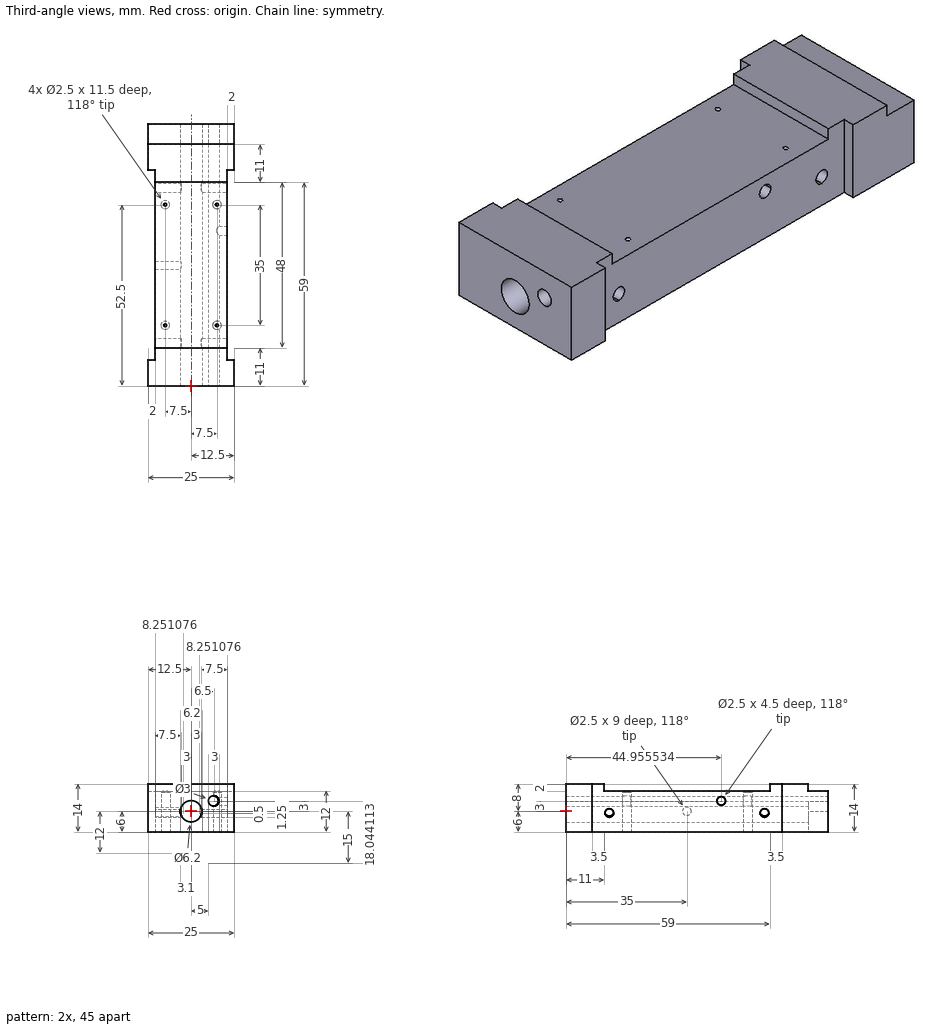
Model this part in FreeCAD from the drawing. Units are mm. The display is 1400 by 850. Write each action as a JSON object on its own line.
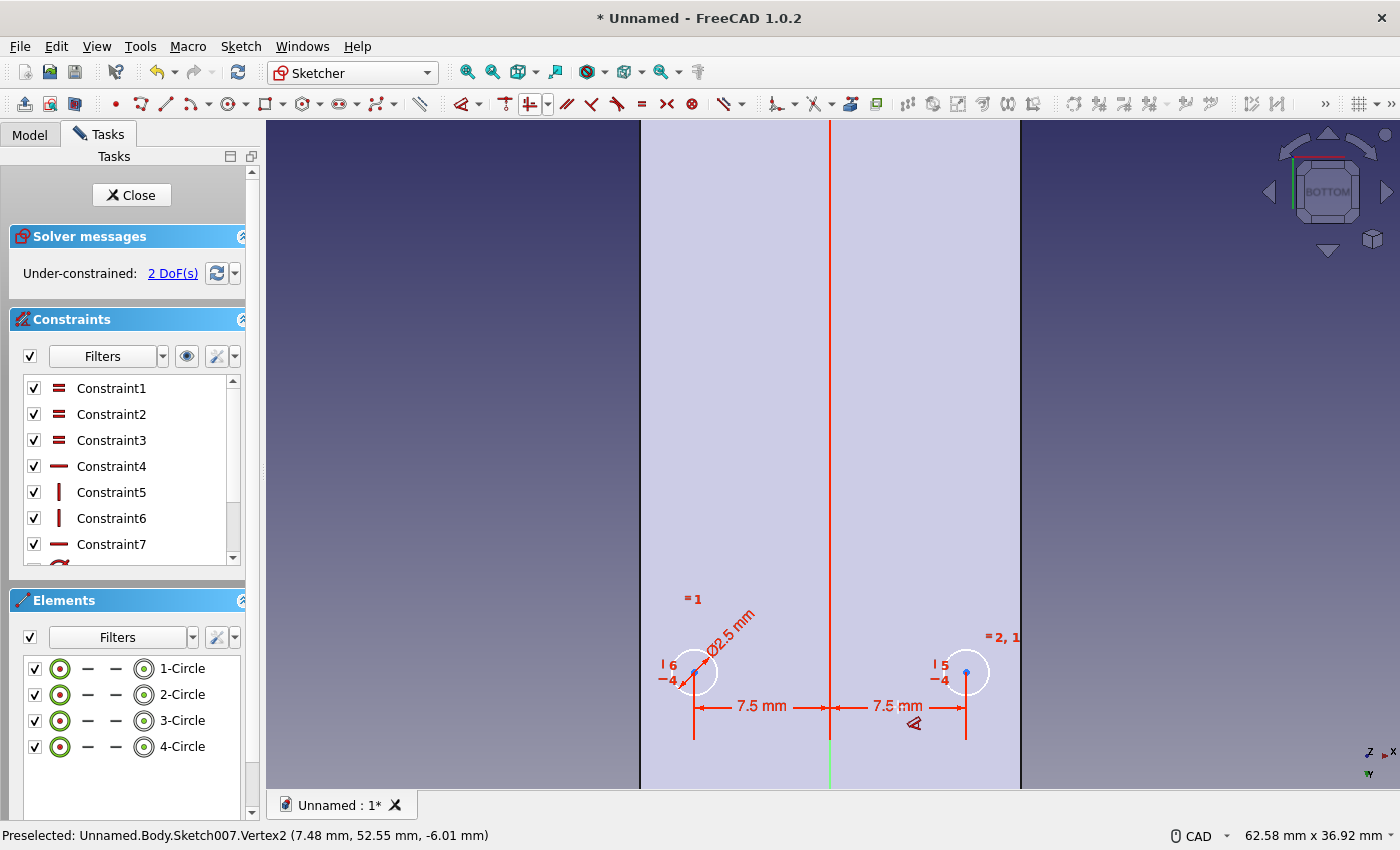
{"action": "left_click", "coordinate": [966, 673]}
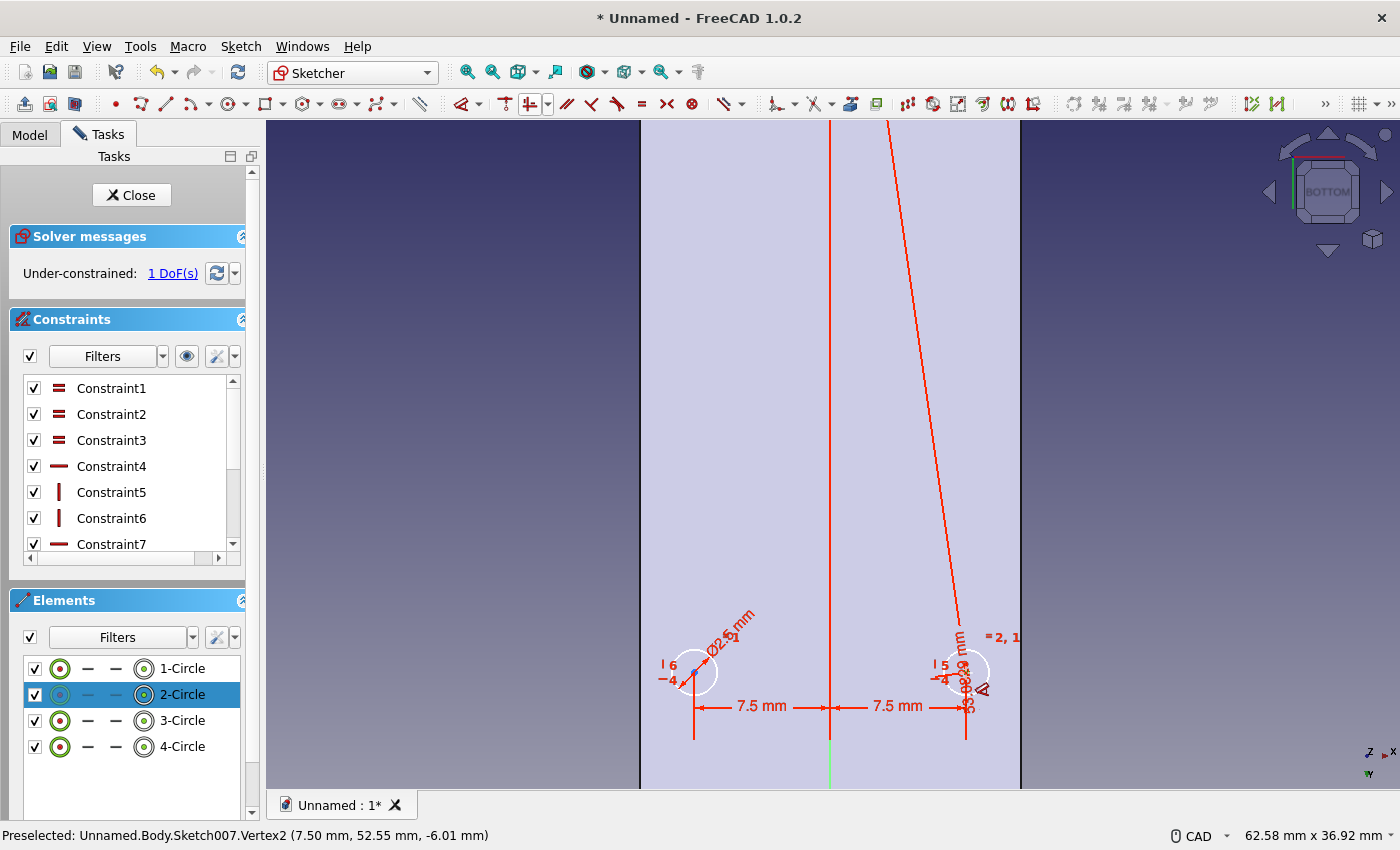
{"action": "scroll", "coordinate": [711, 656], "scroll_direction": "down", "scroll_amount": 4}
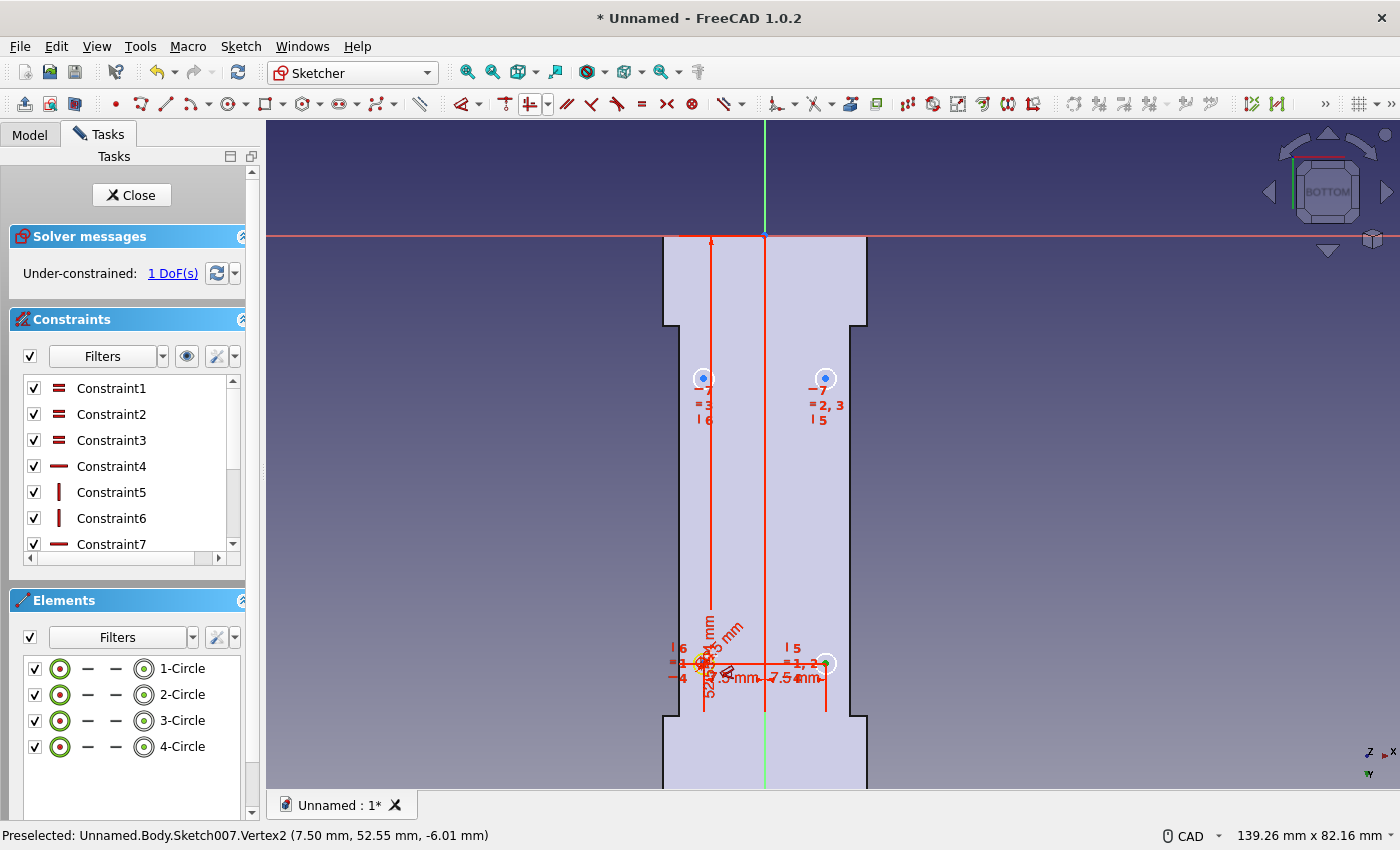
{"action": "left_click", "coordinate": [826, 379]}
{"action": "left_click", "coordinate": [860, 521]}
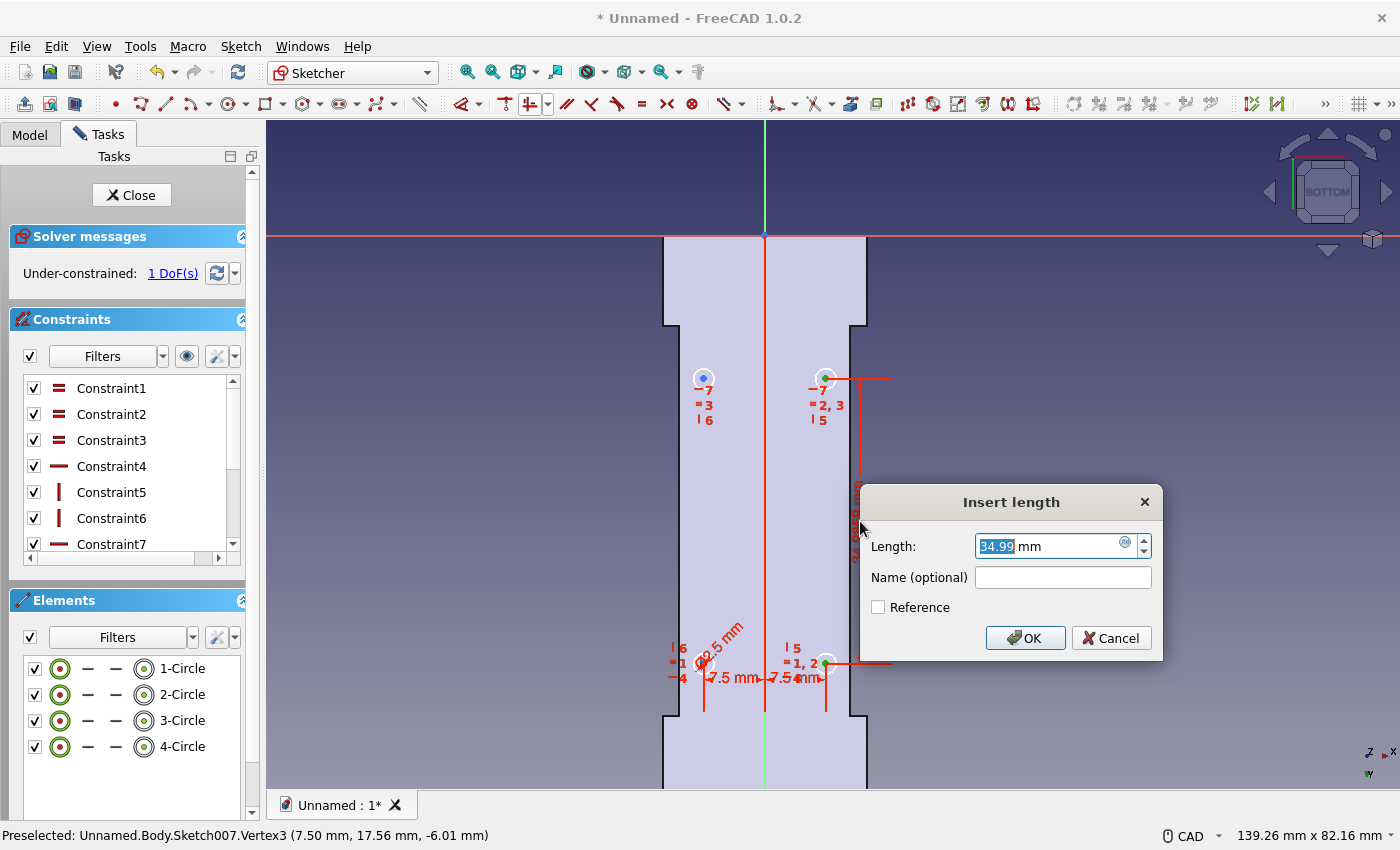
{"action": "type", "text": "35"}
{"action": "key", "text": "Return"}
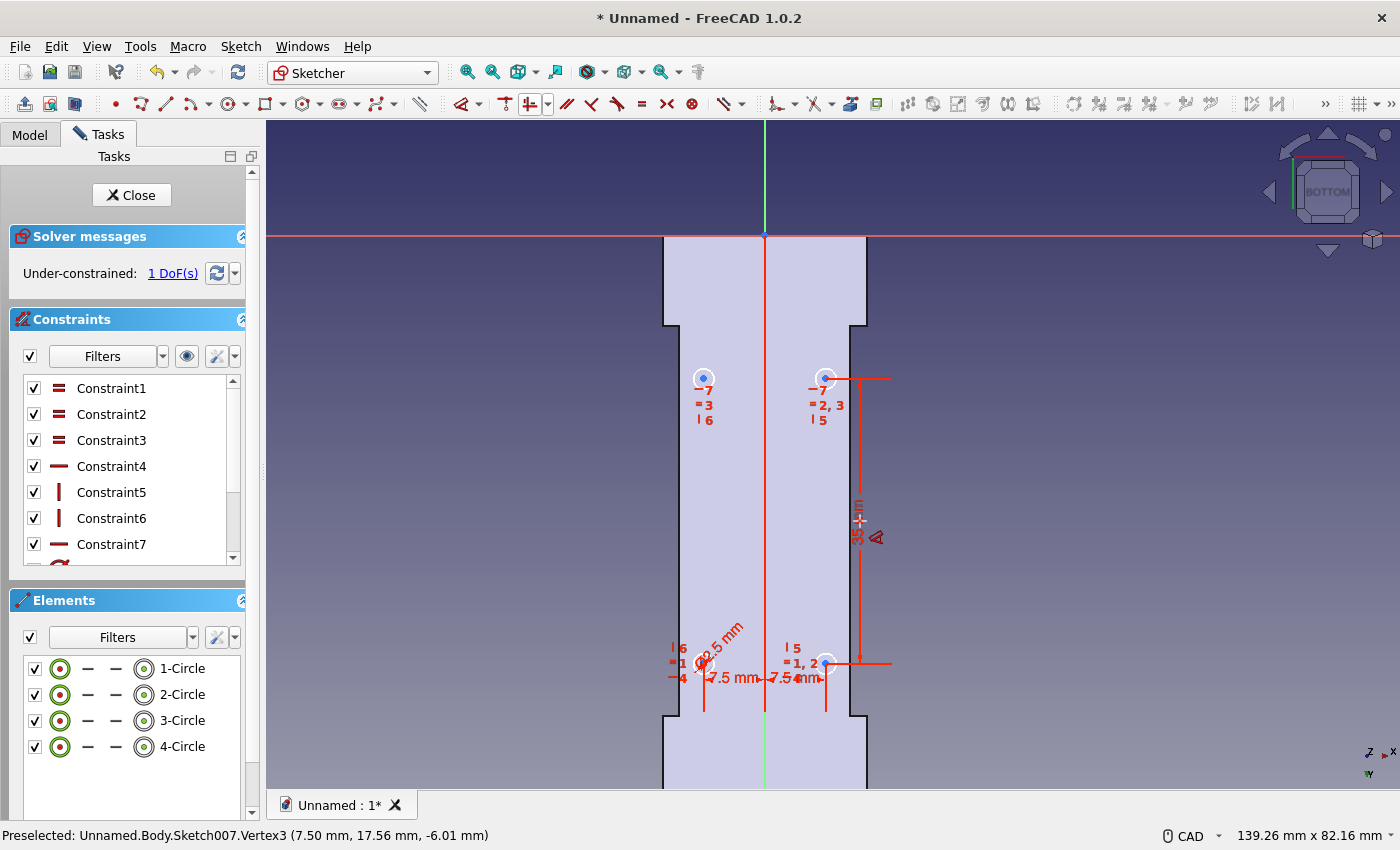
{"action": "left_click", "coordinate": [704, 664]}
{"action": "left_click", "coordinate": [670, 450]}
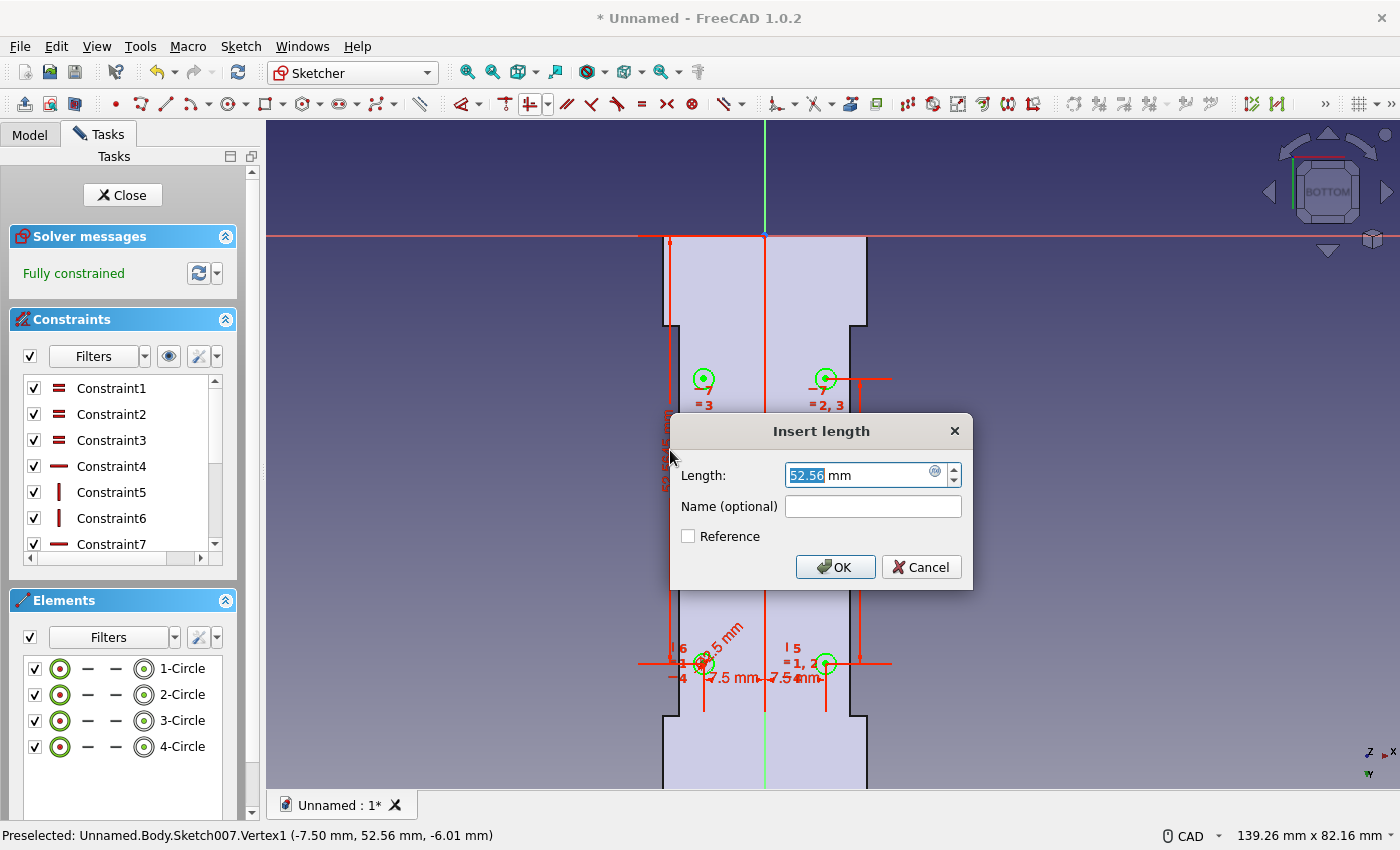
{"action": "type", "text": "52.5"}
{"action": "key", "text": "Return"}
{"action": "key", "text": "Escape"}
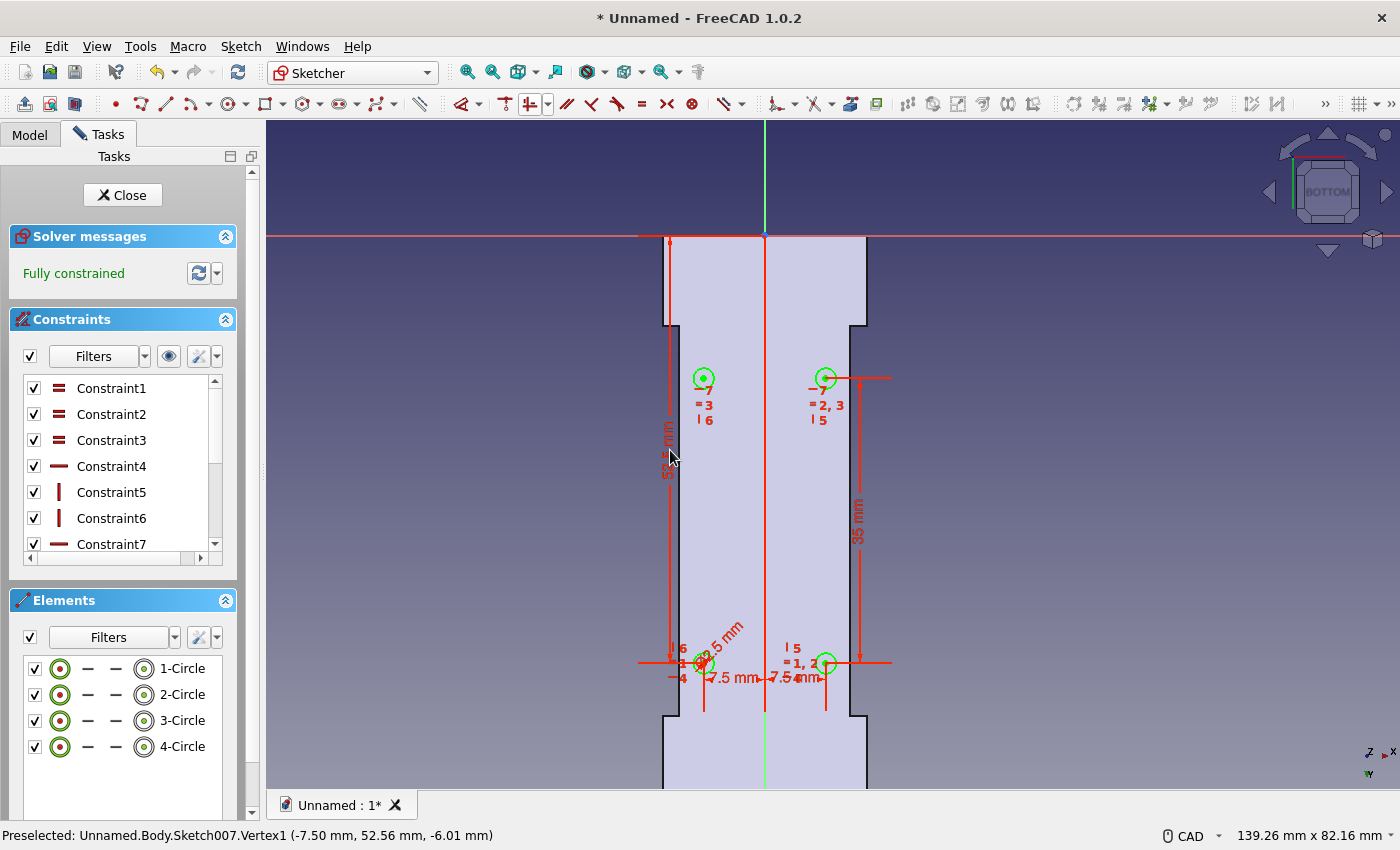
{"action": "left_click", "coordinate": [123, 195]}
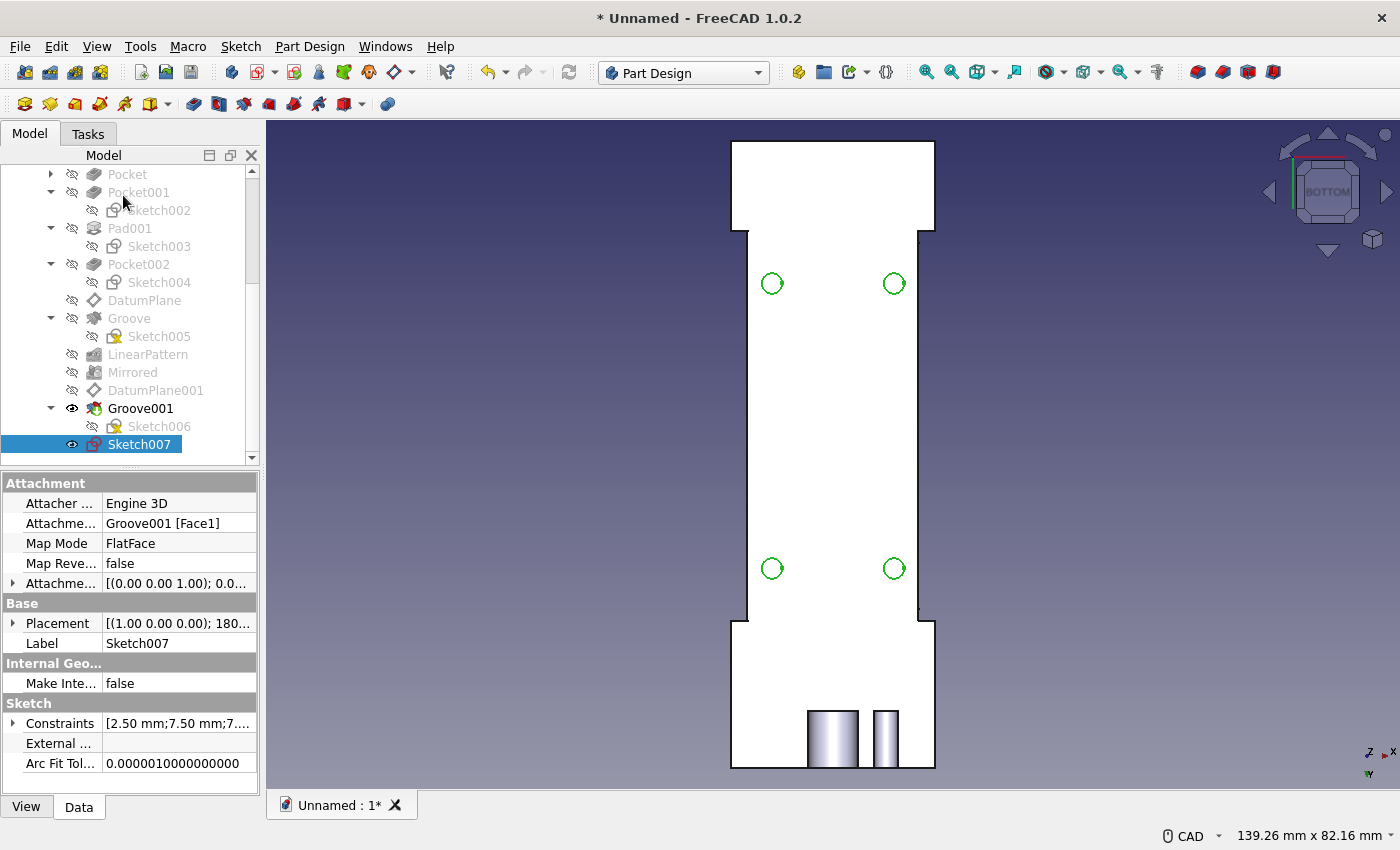
{"action": "left_click", "coordinate": [219, 104]}